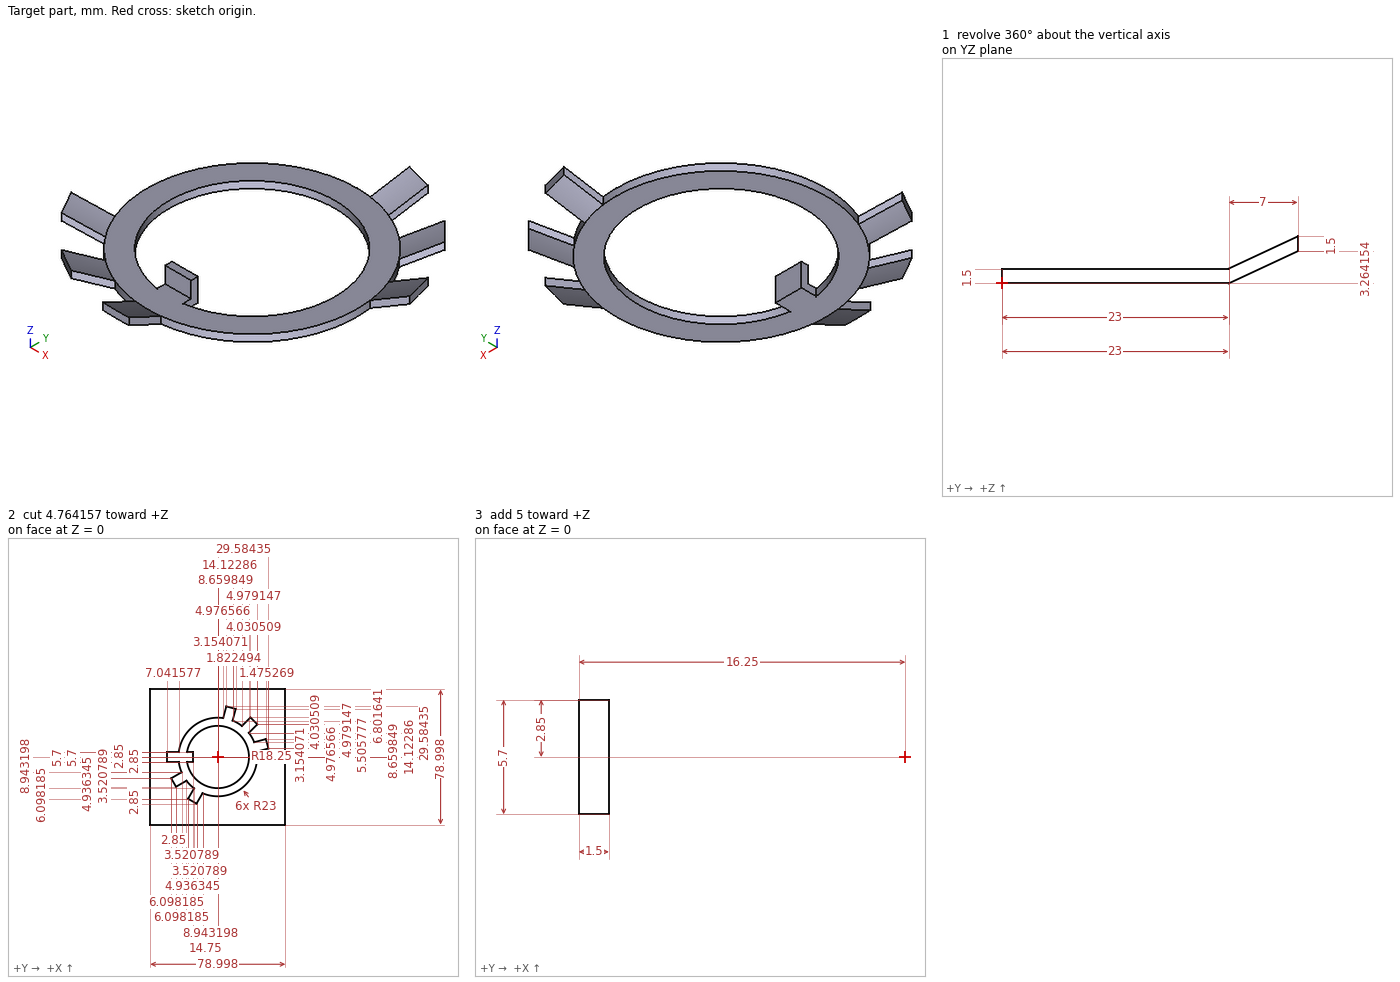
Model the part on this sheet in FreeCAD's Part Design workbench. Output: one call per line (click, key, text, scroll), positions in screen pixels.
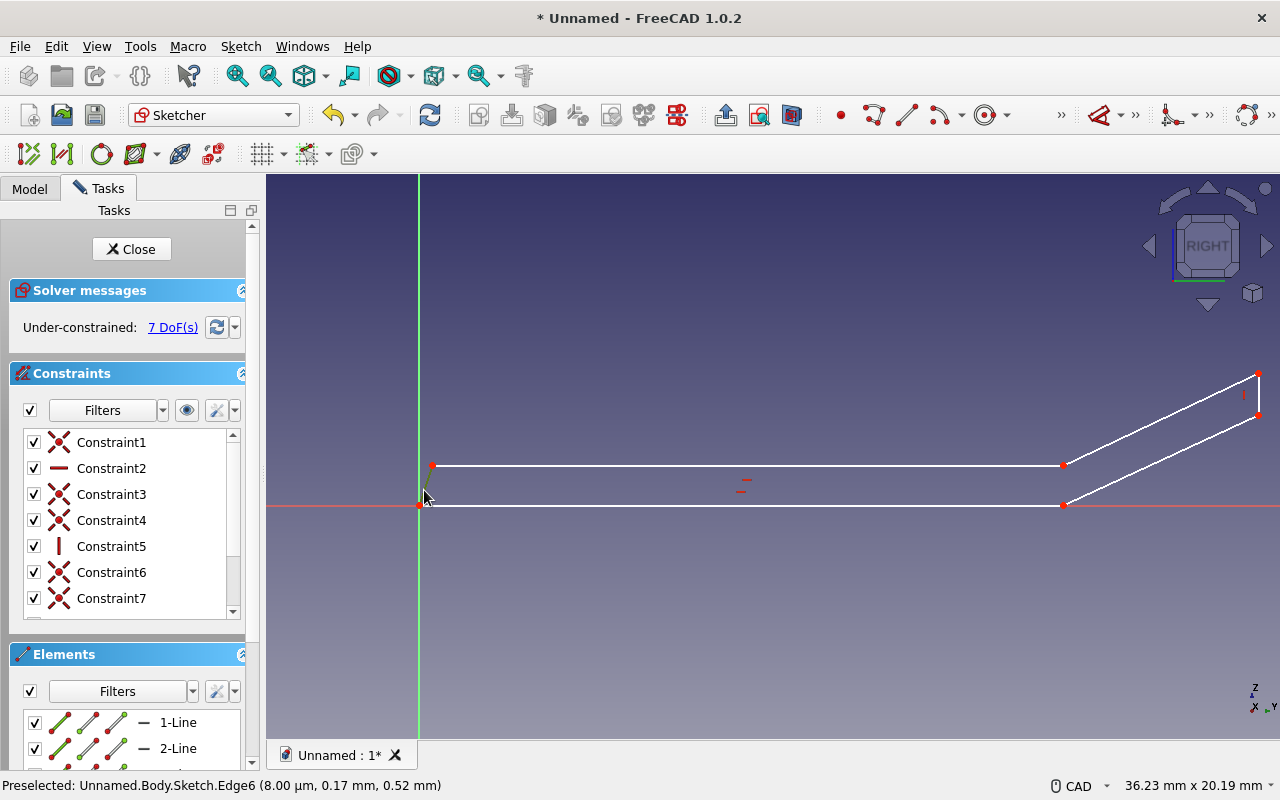
key(v)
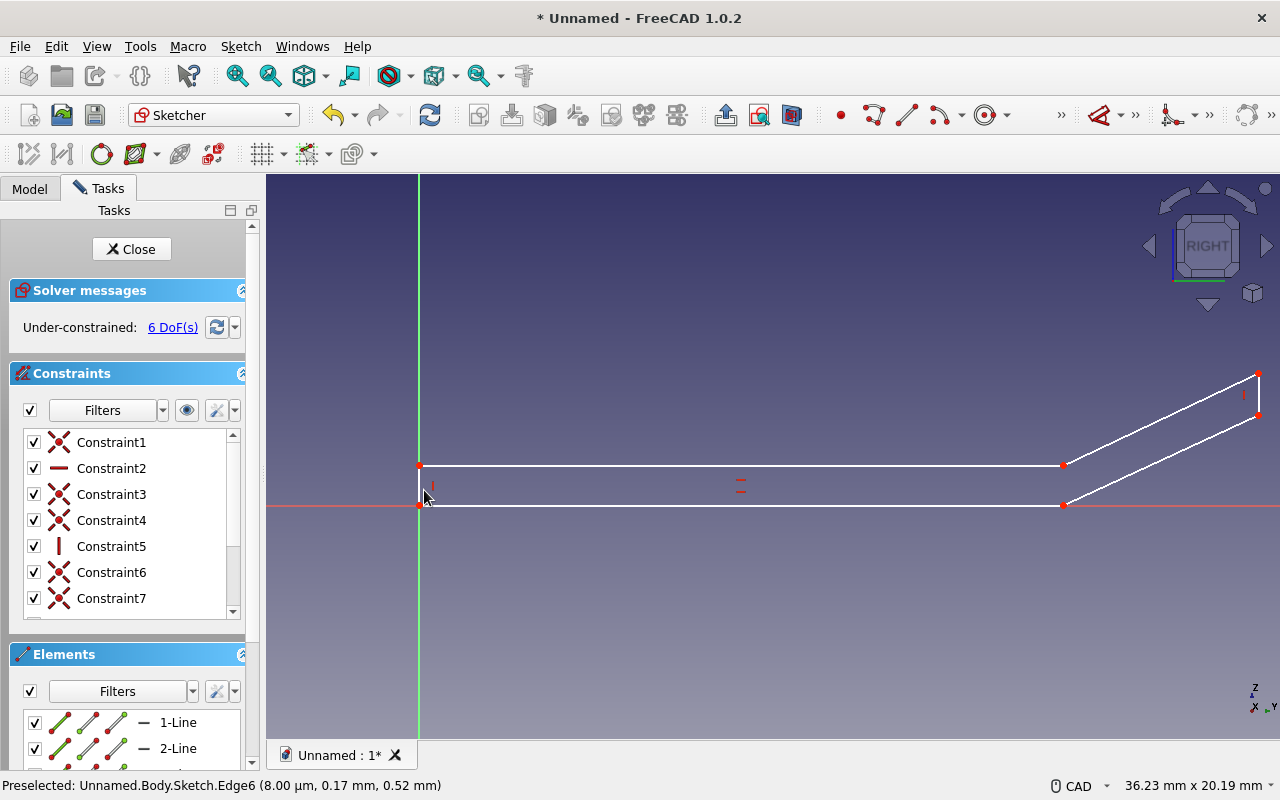
click(612, 506)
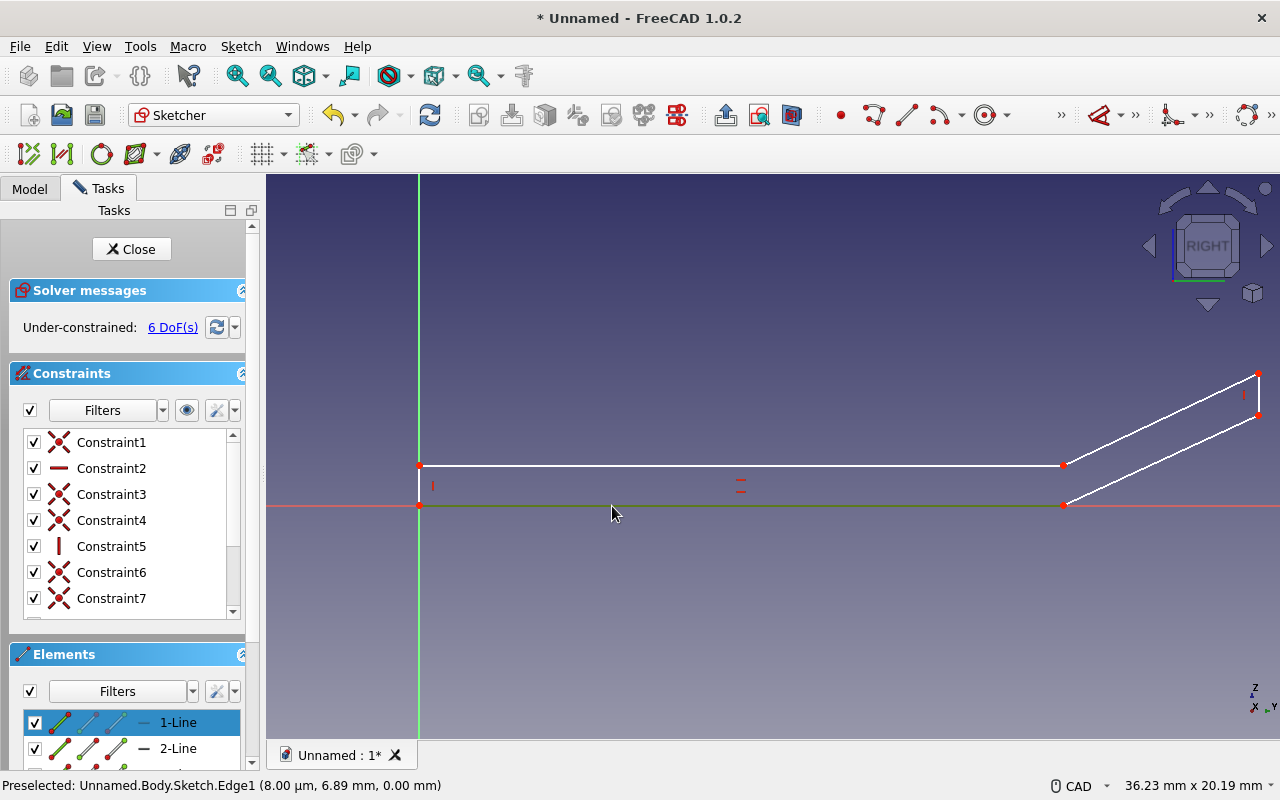
key(l)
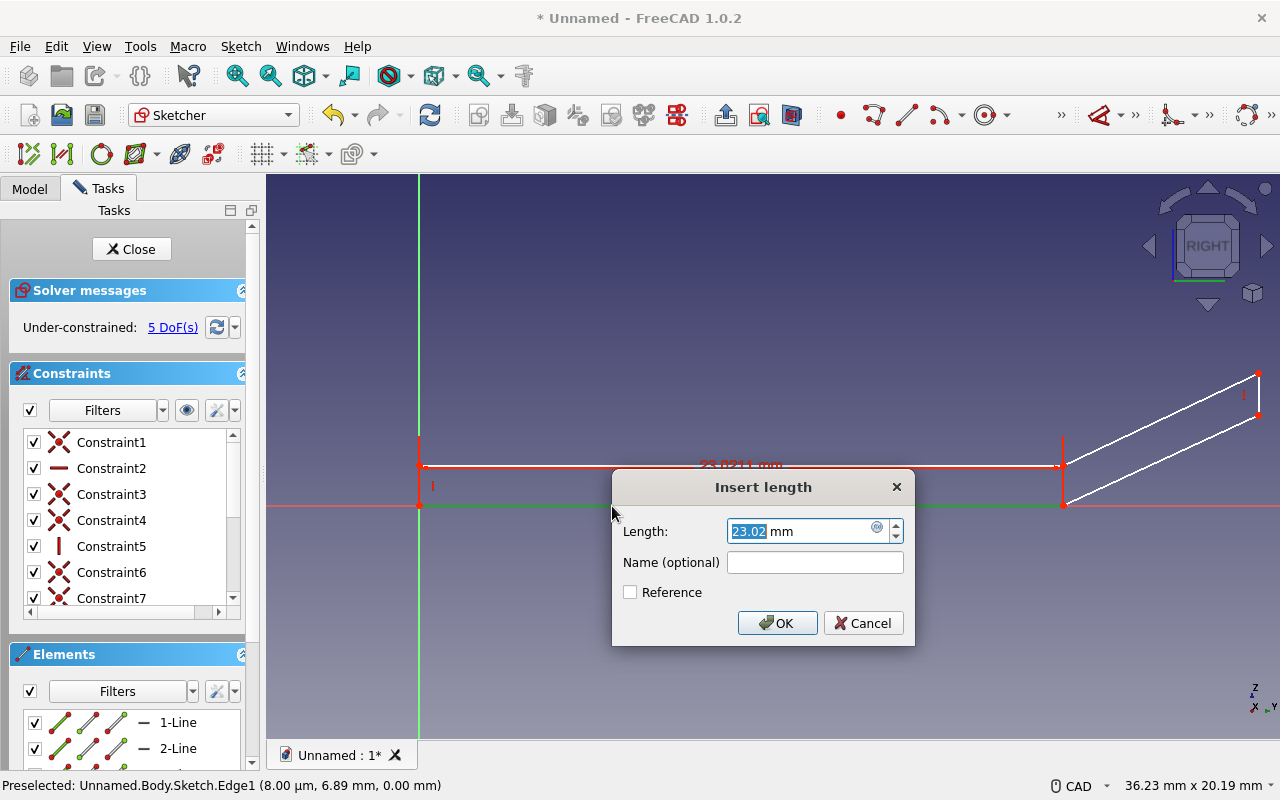
text(23)
key(Return)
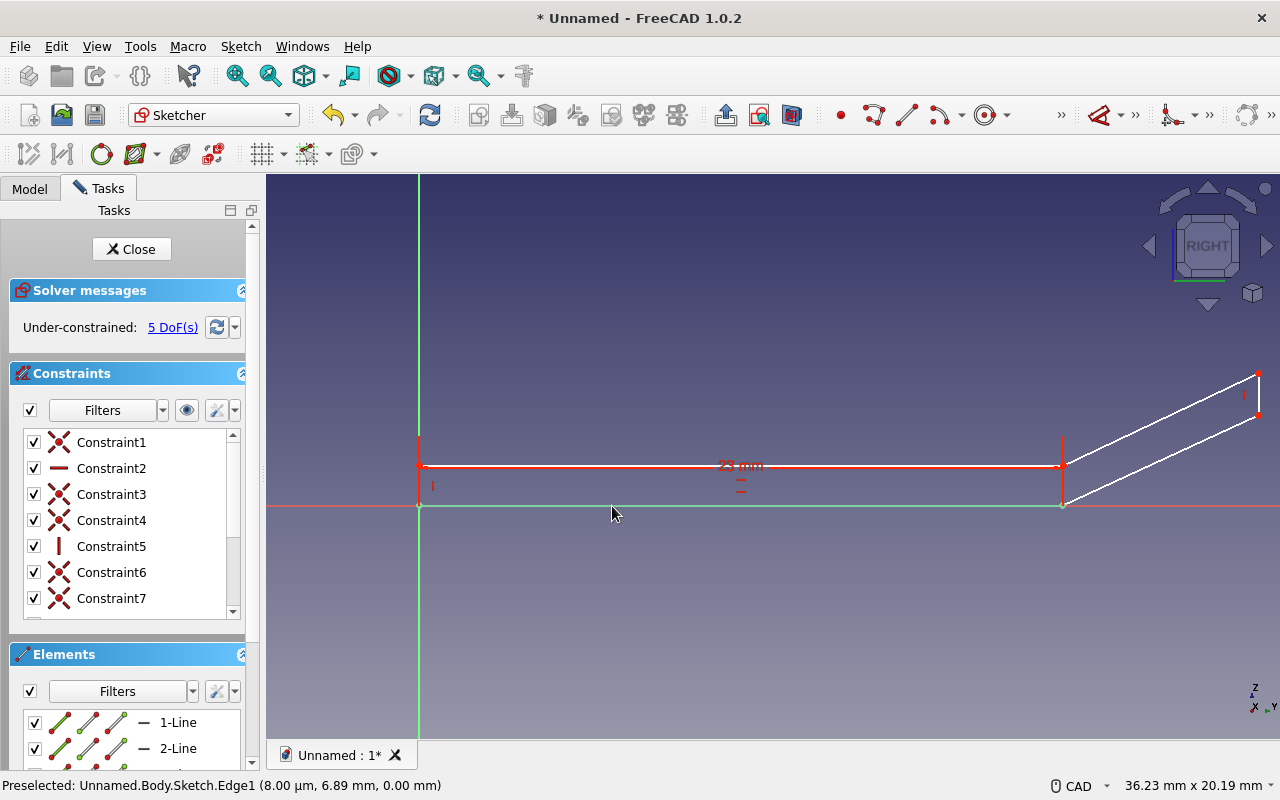
click(870, 466)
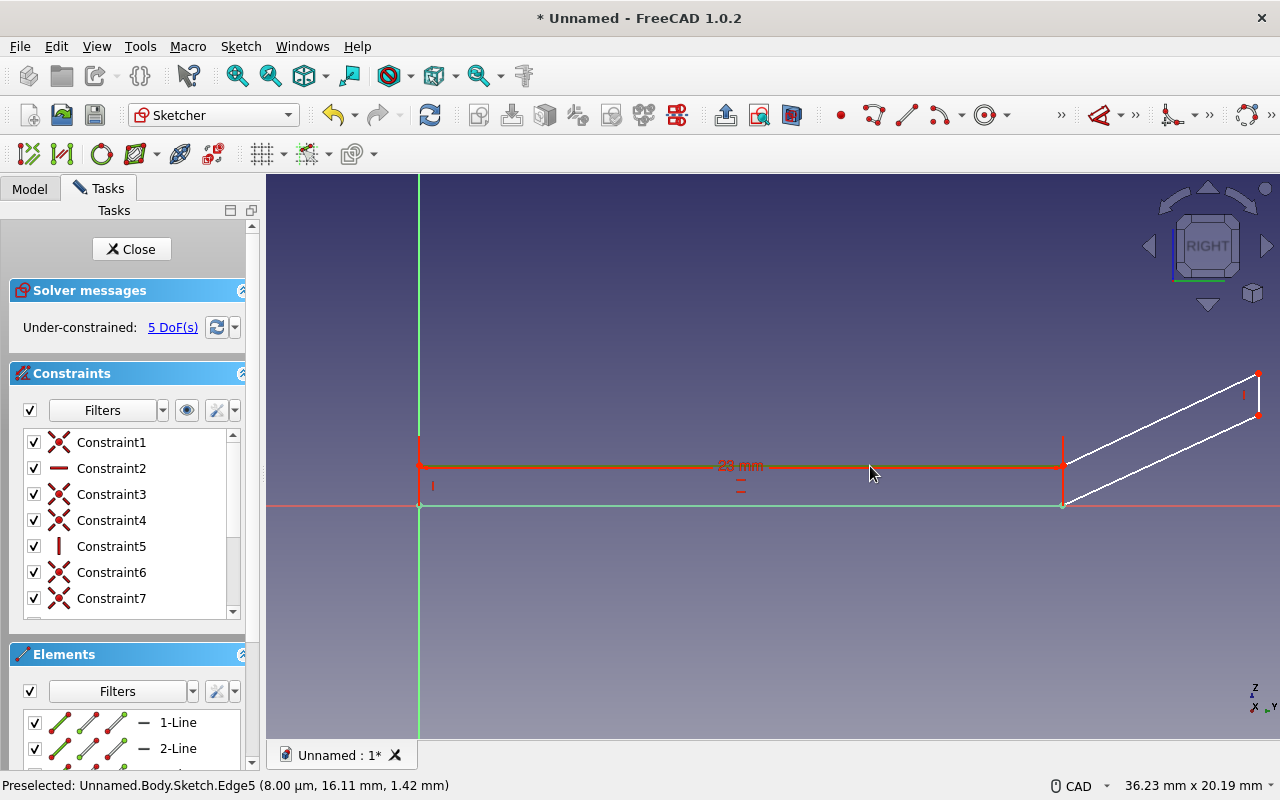
key(l)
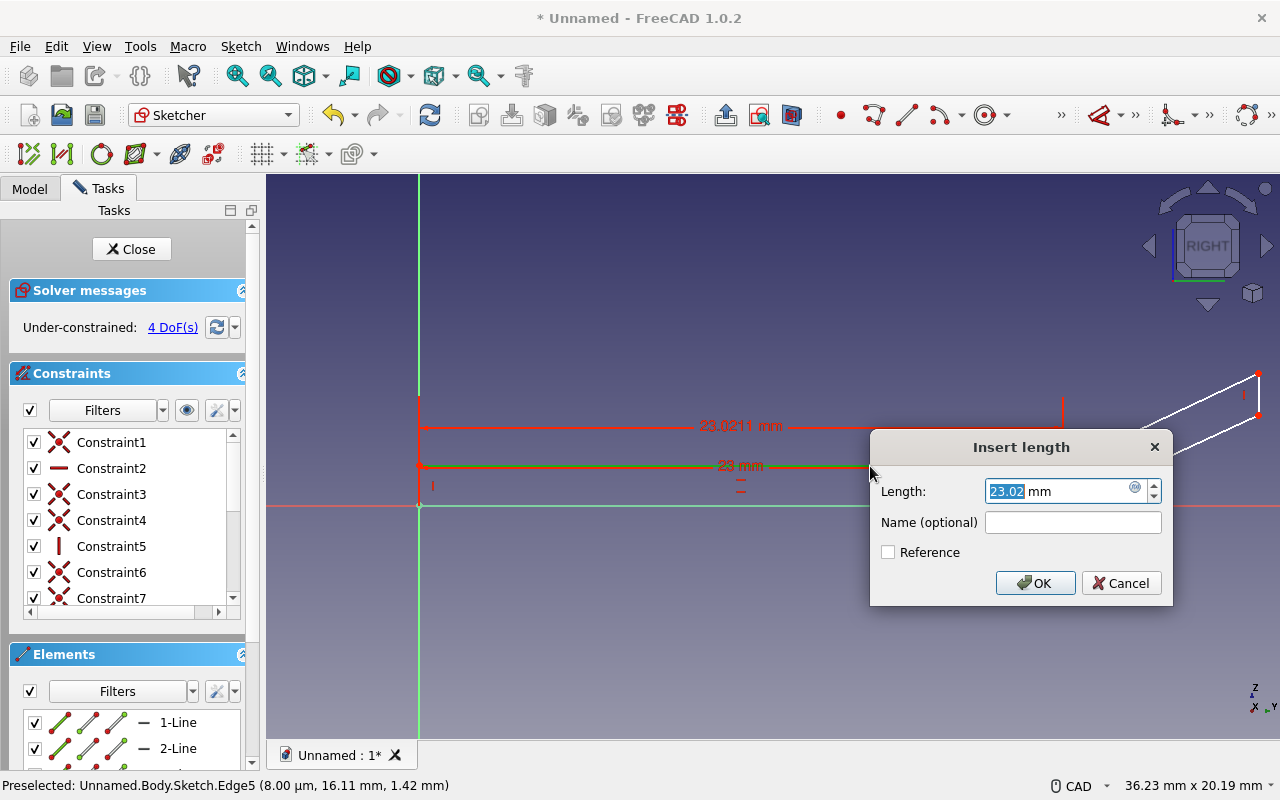
text(23)
key(Return)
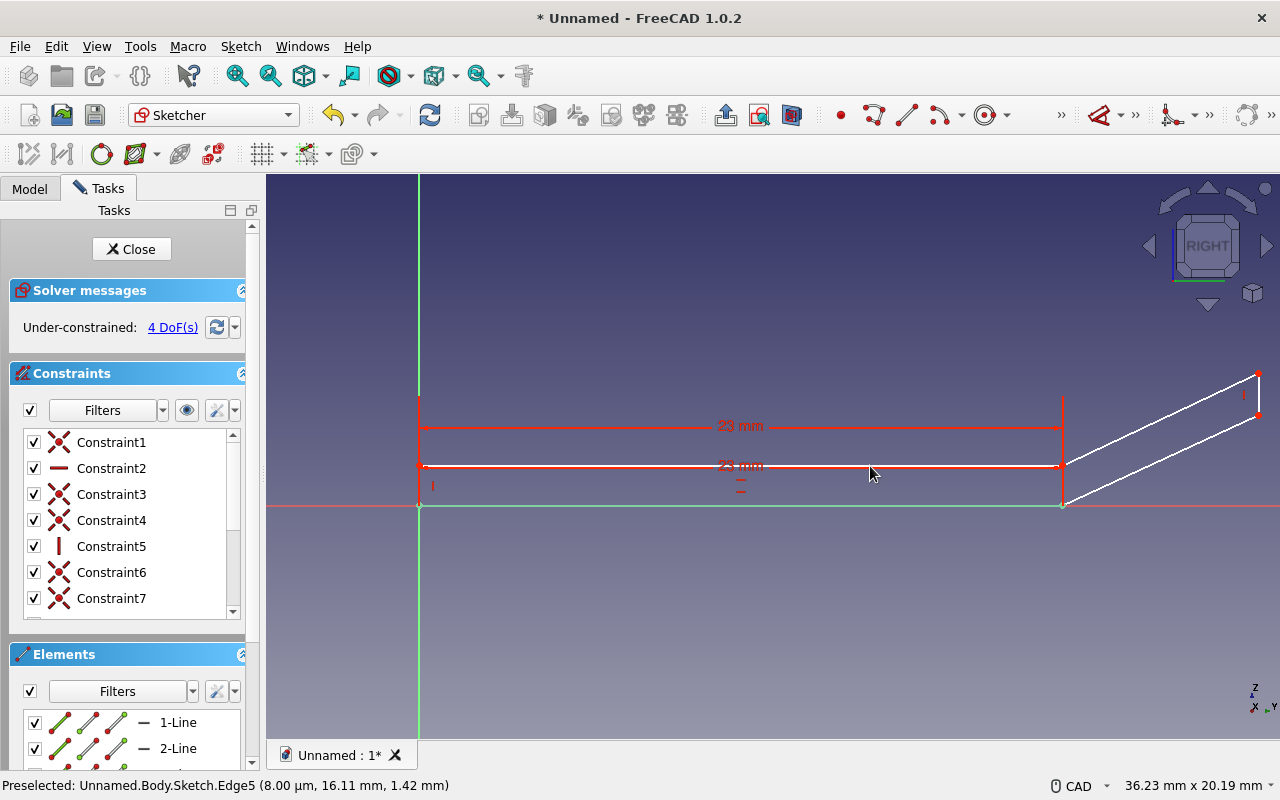
click(1102, 488)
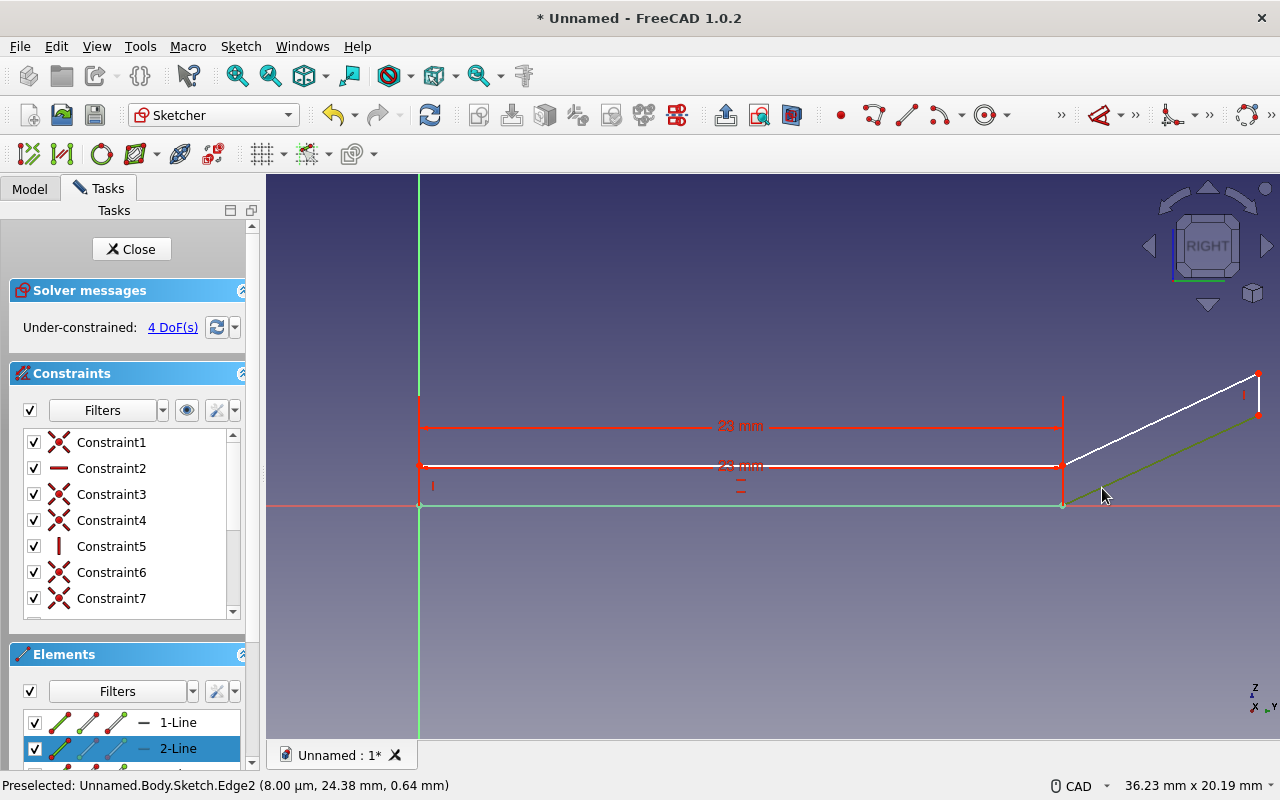
click(1120, 116)